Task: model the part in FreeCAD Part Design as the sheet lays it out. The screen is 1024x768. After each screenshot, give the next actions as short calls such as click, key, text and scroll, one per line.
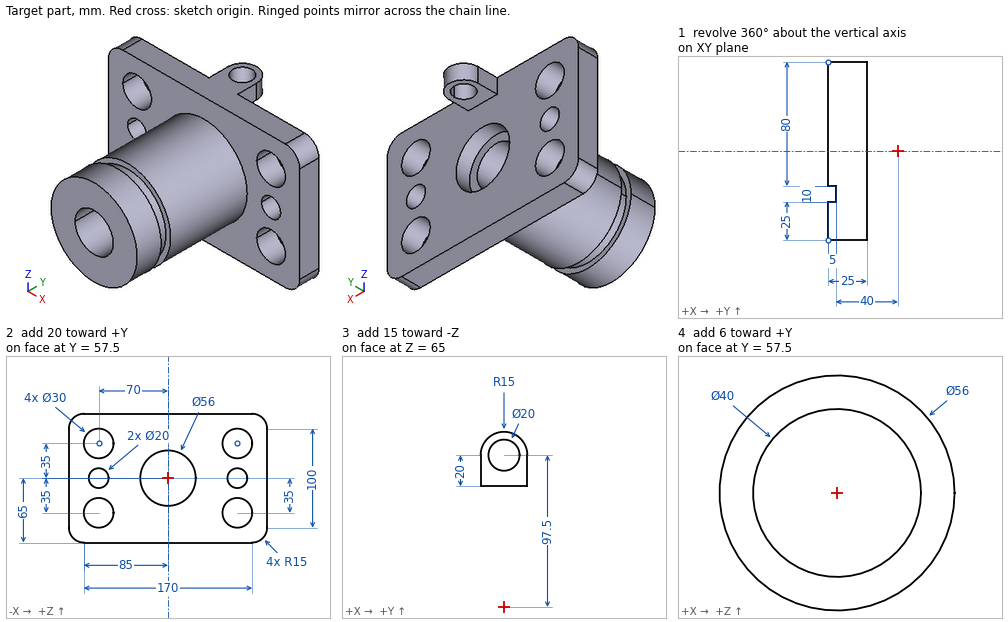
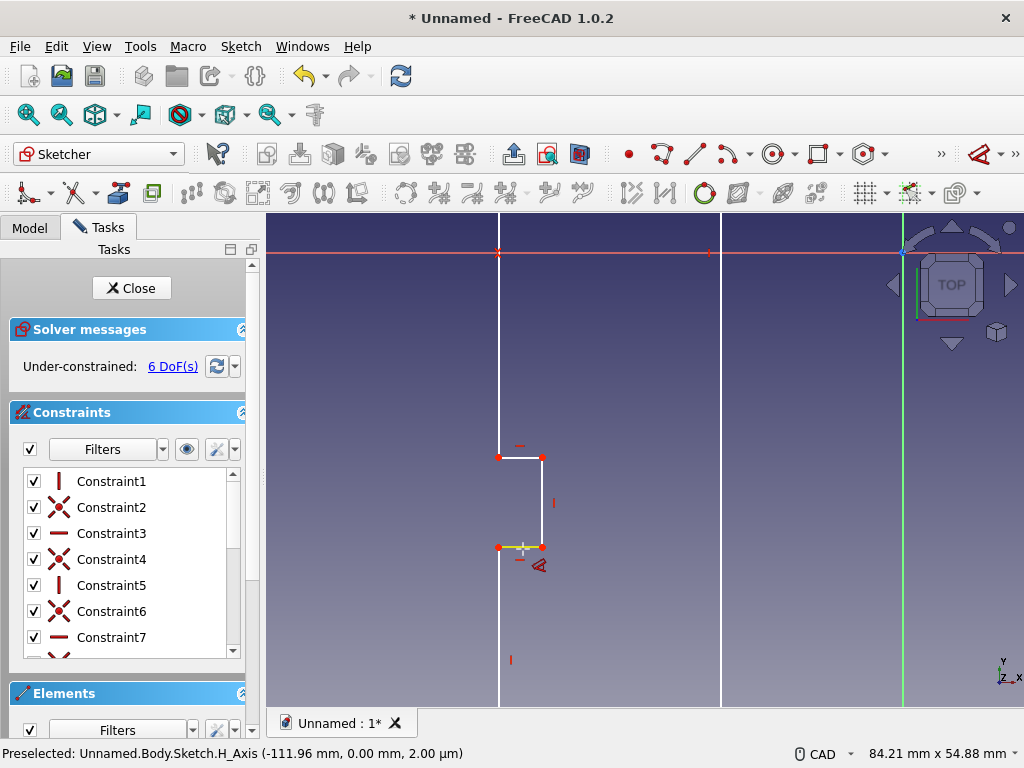
click(521, 547)
click(521, 581)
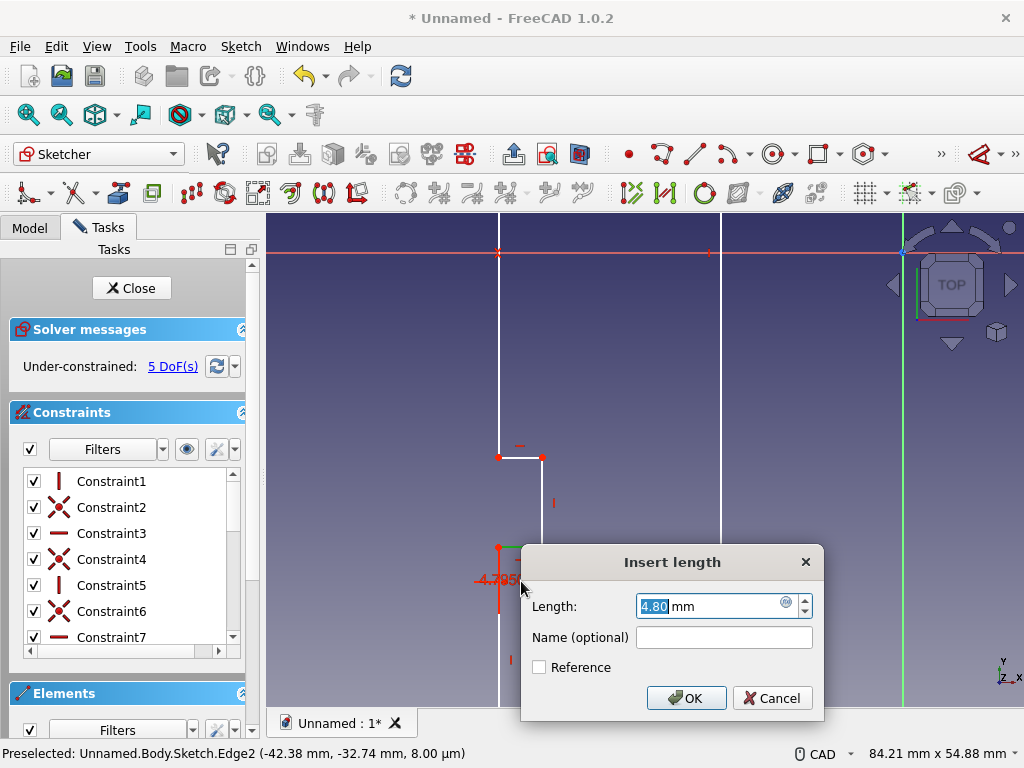
text(5)
key(Return)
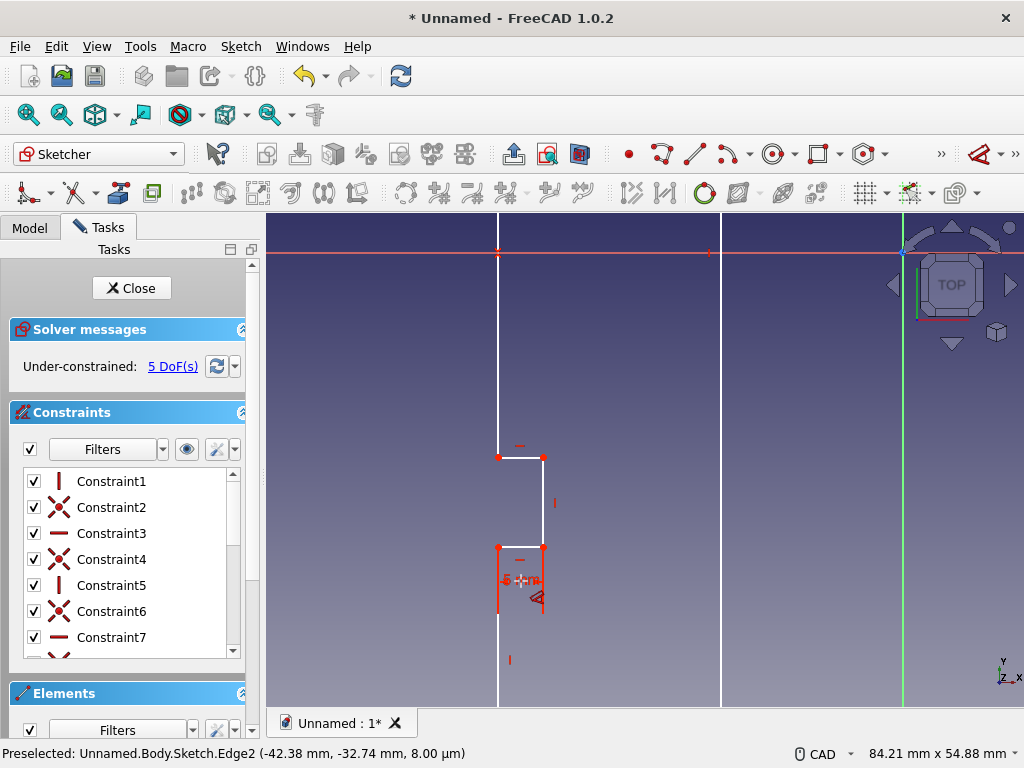
click(543, 485)
click(509, 503)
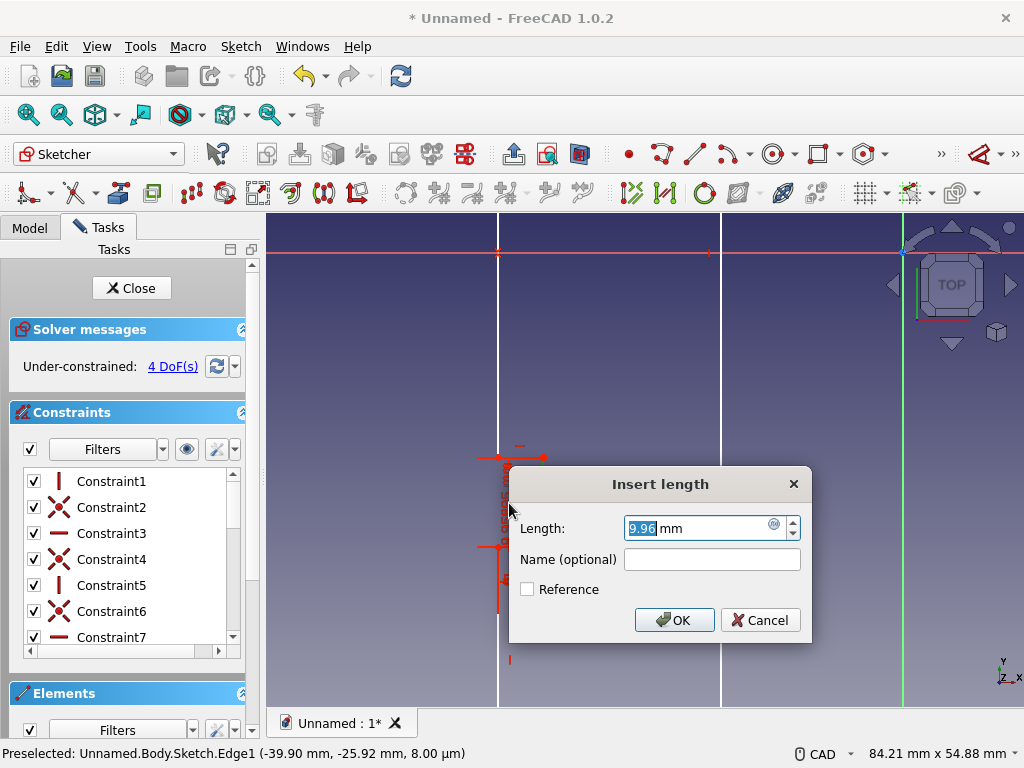
text(10)
key(Return)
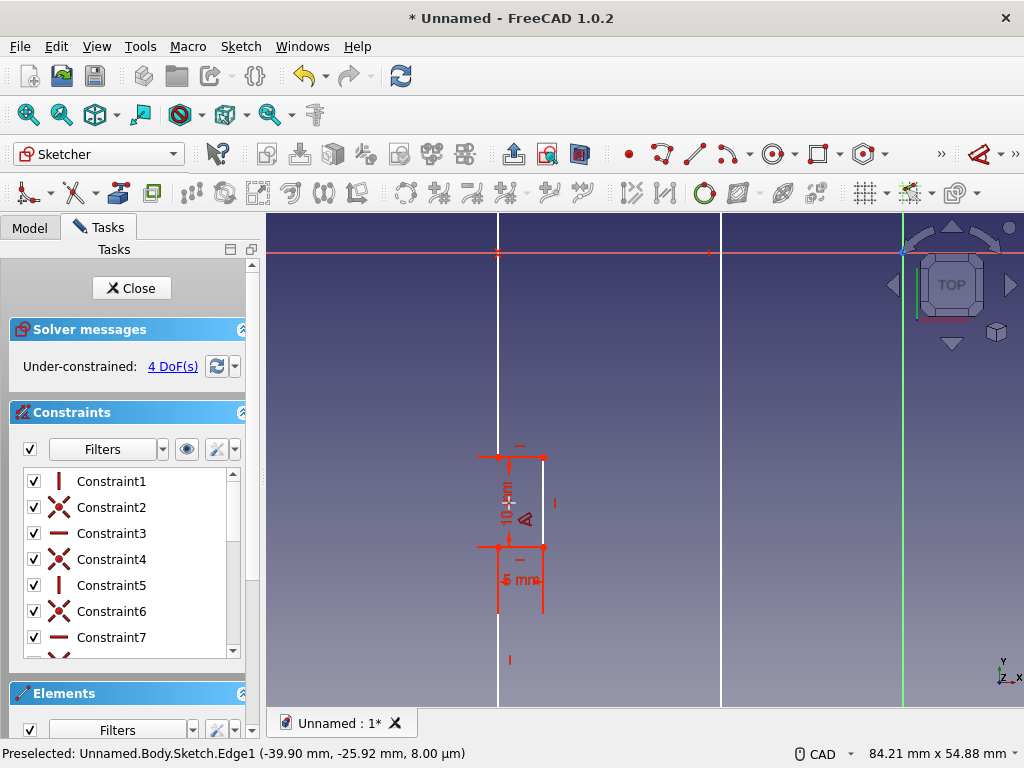
click(498, 614)
click(464, 613)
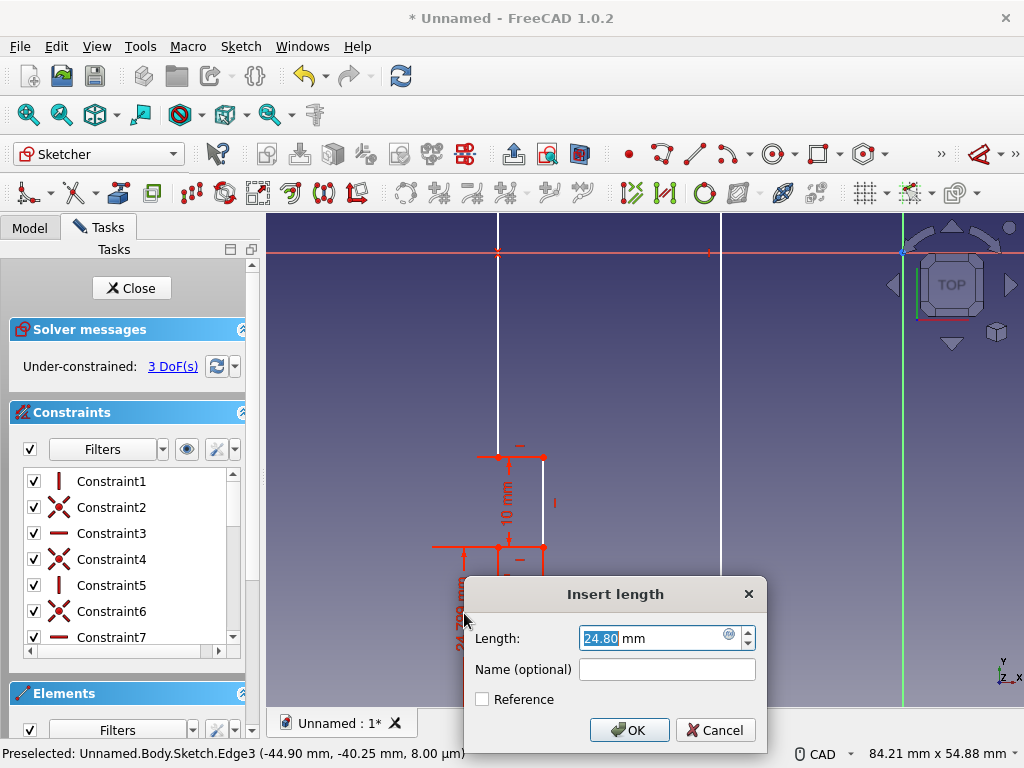
text(25)
key(Return)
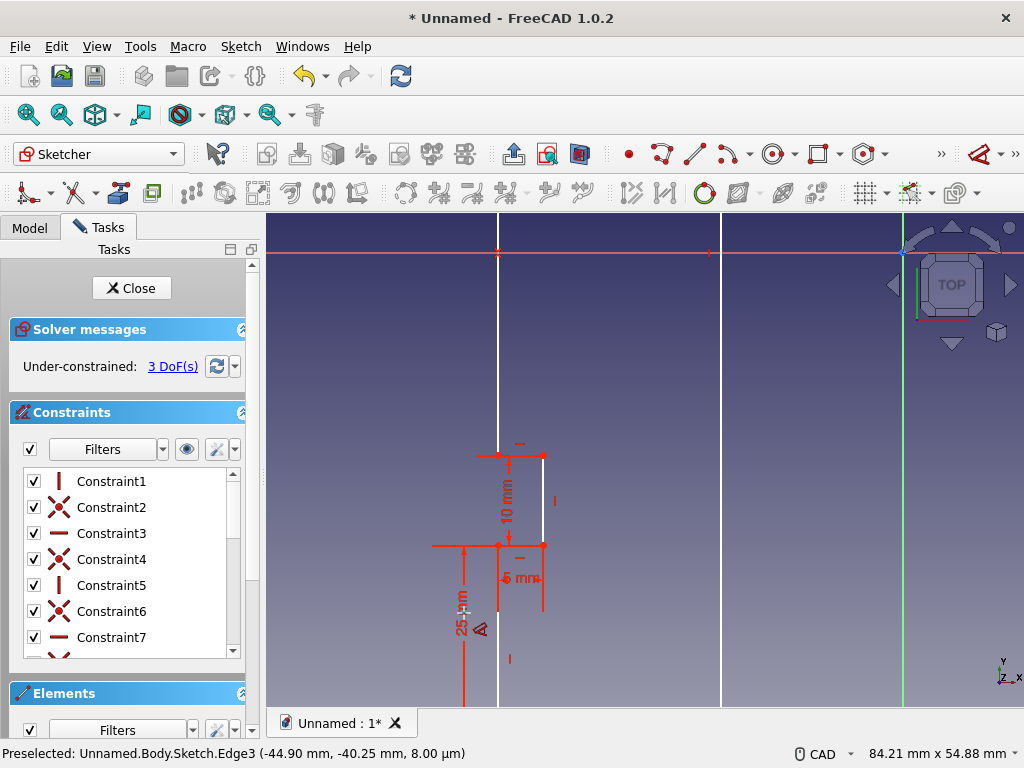
scroll(523, 549, down, 6)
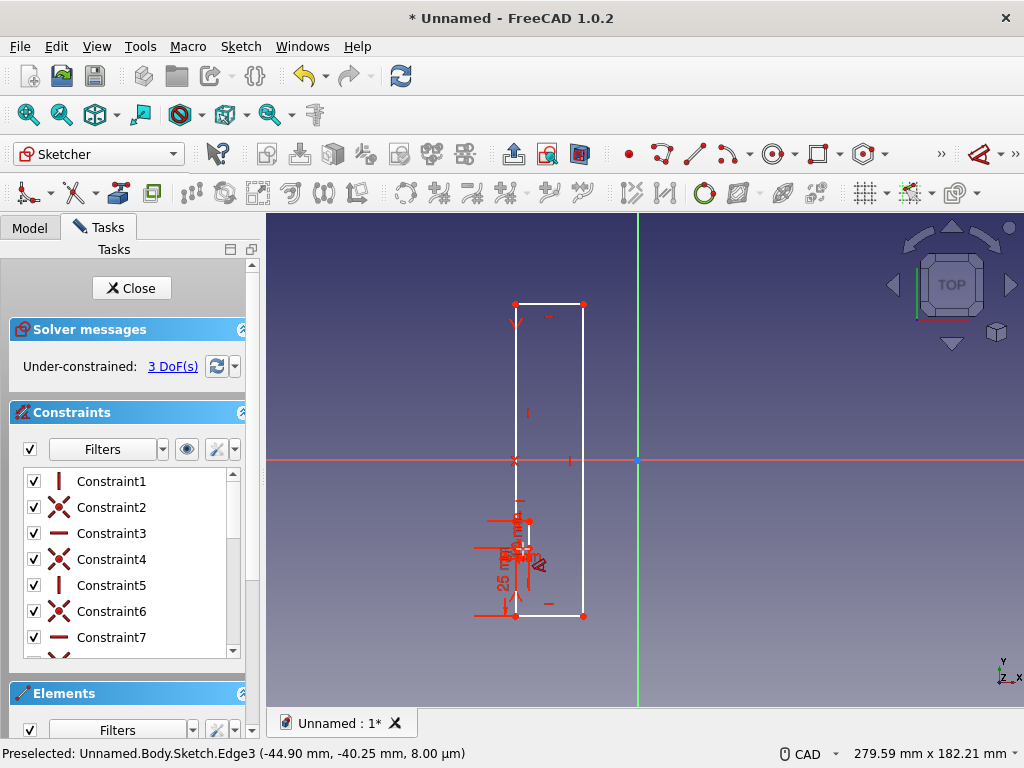
click(536, 616)
click(549, 650)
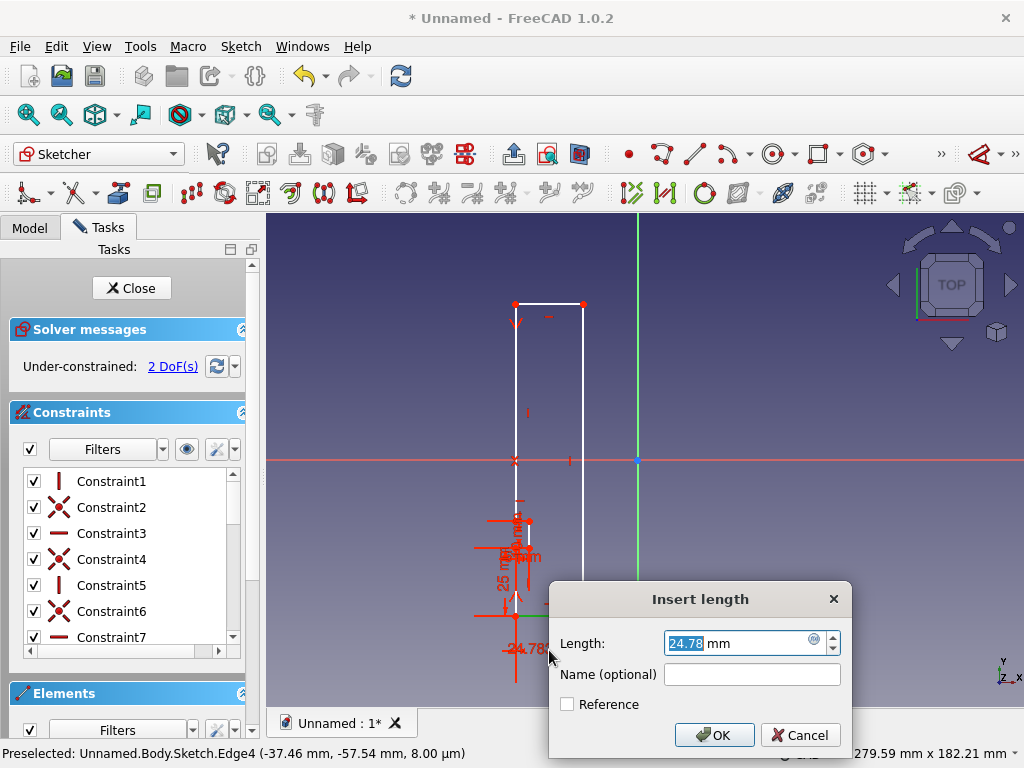
text(25)
key(Return)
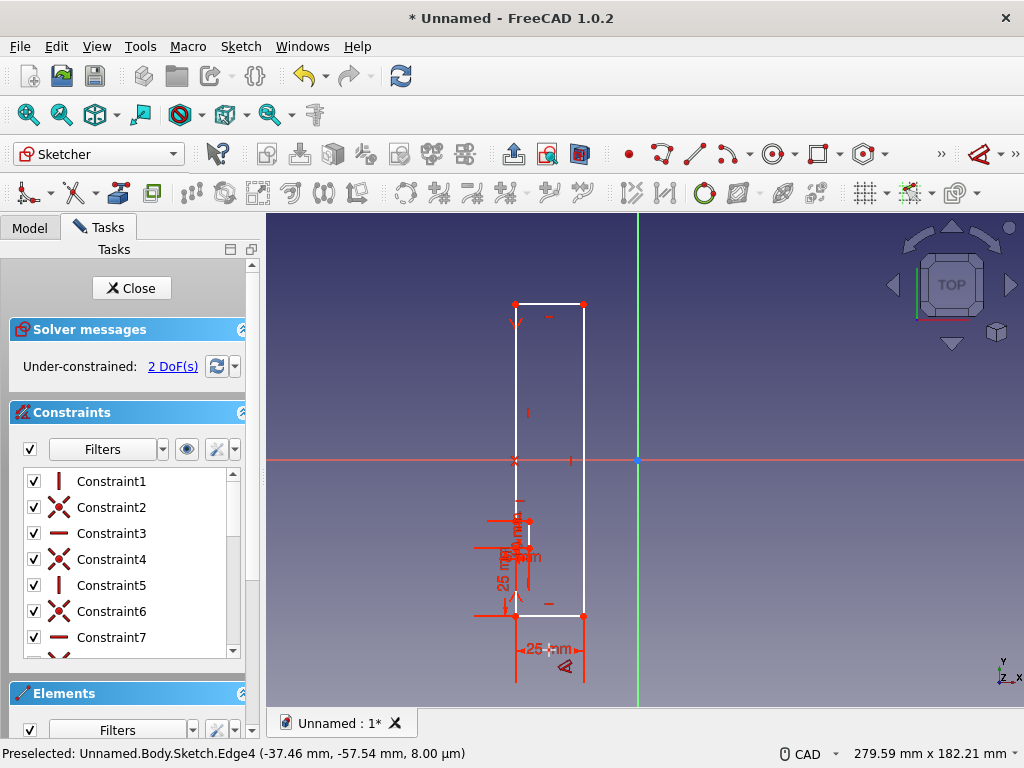
click(516, 369)
click(482, 413)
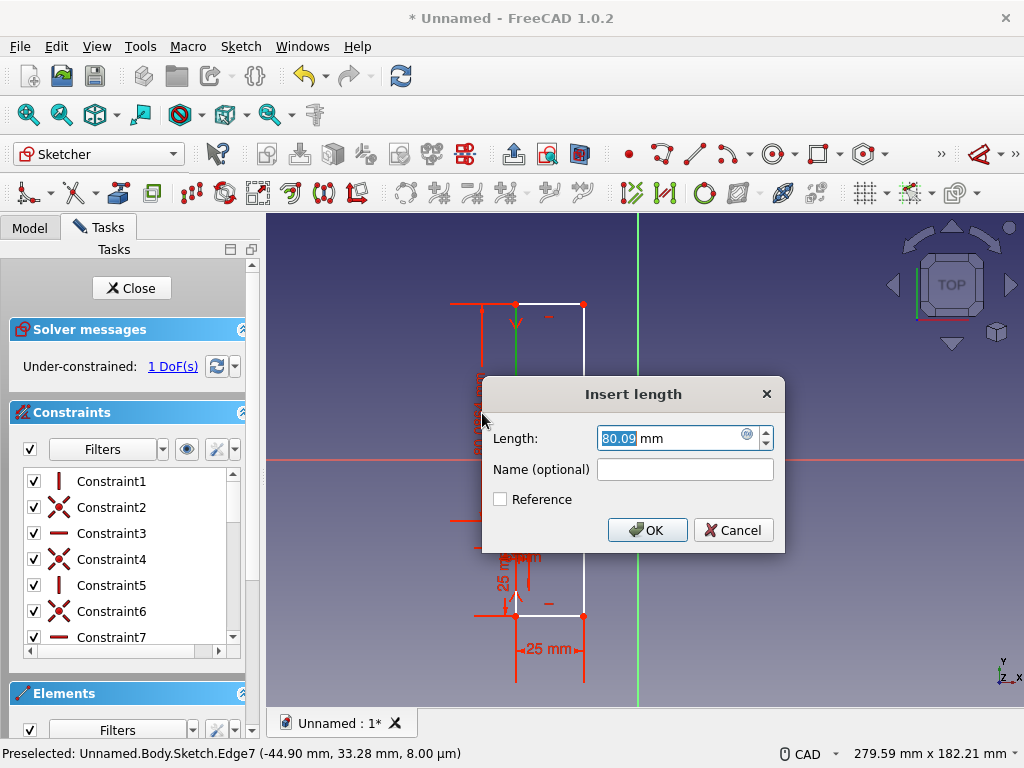
text(80)
key(Return)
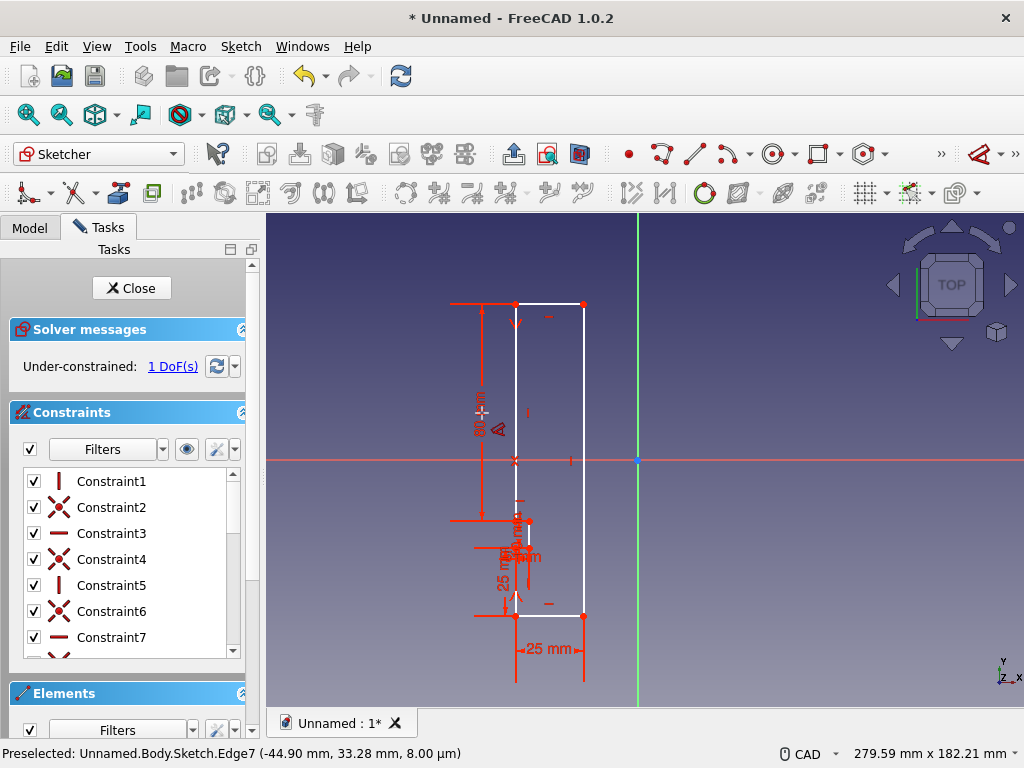
click(529, 521)
click(608, 555)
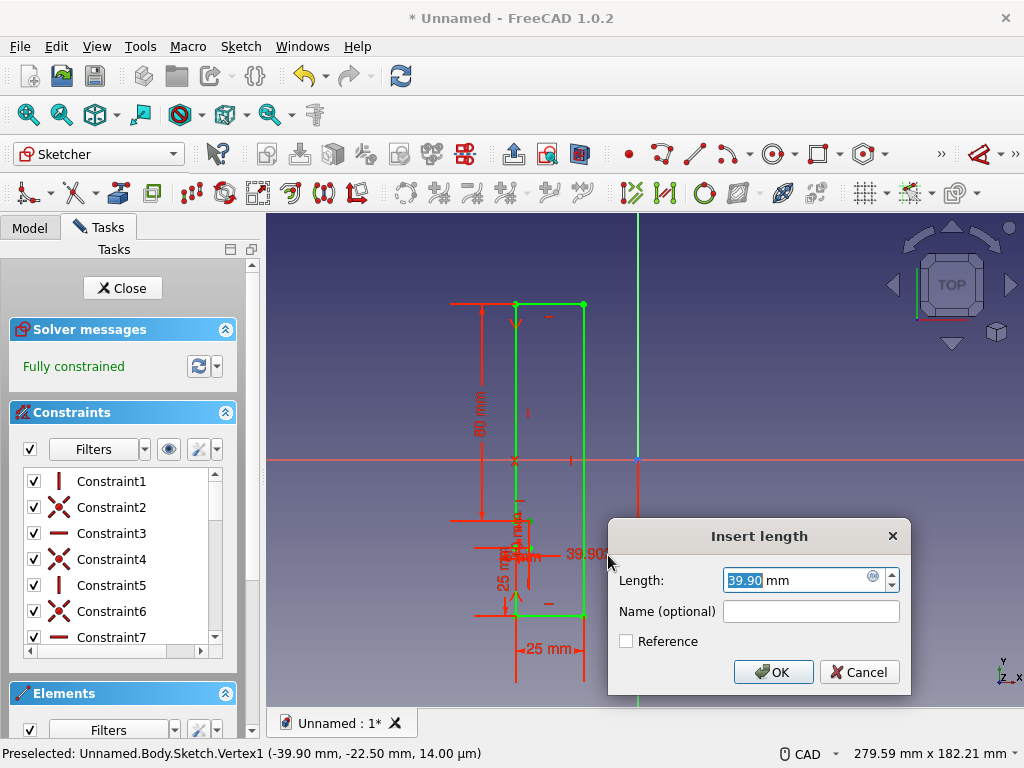
text(40)
key(Return)
key(Escape)